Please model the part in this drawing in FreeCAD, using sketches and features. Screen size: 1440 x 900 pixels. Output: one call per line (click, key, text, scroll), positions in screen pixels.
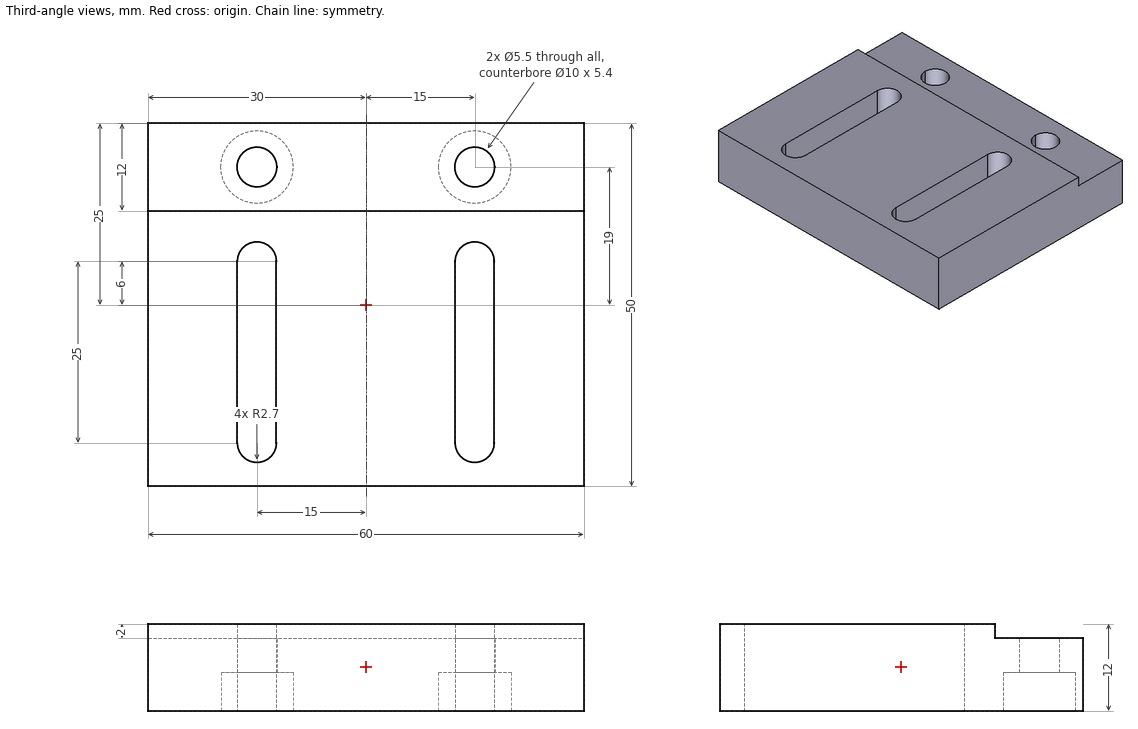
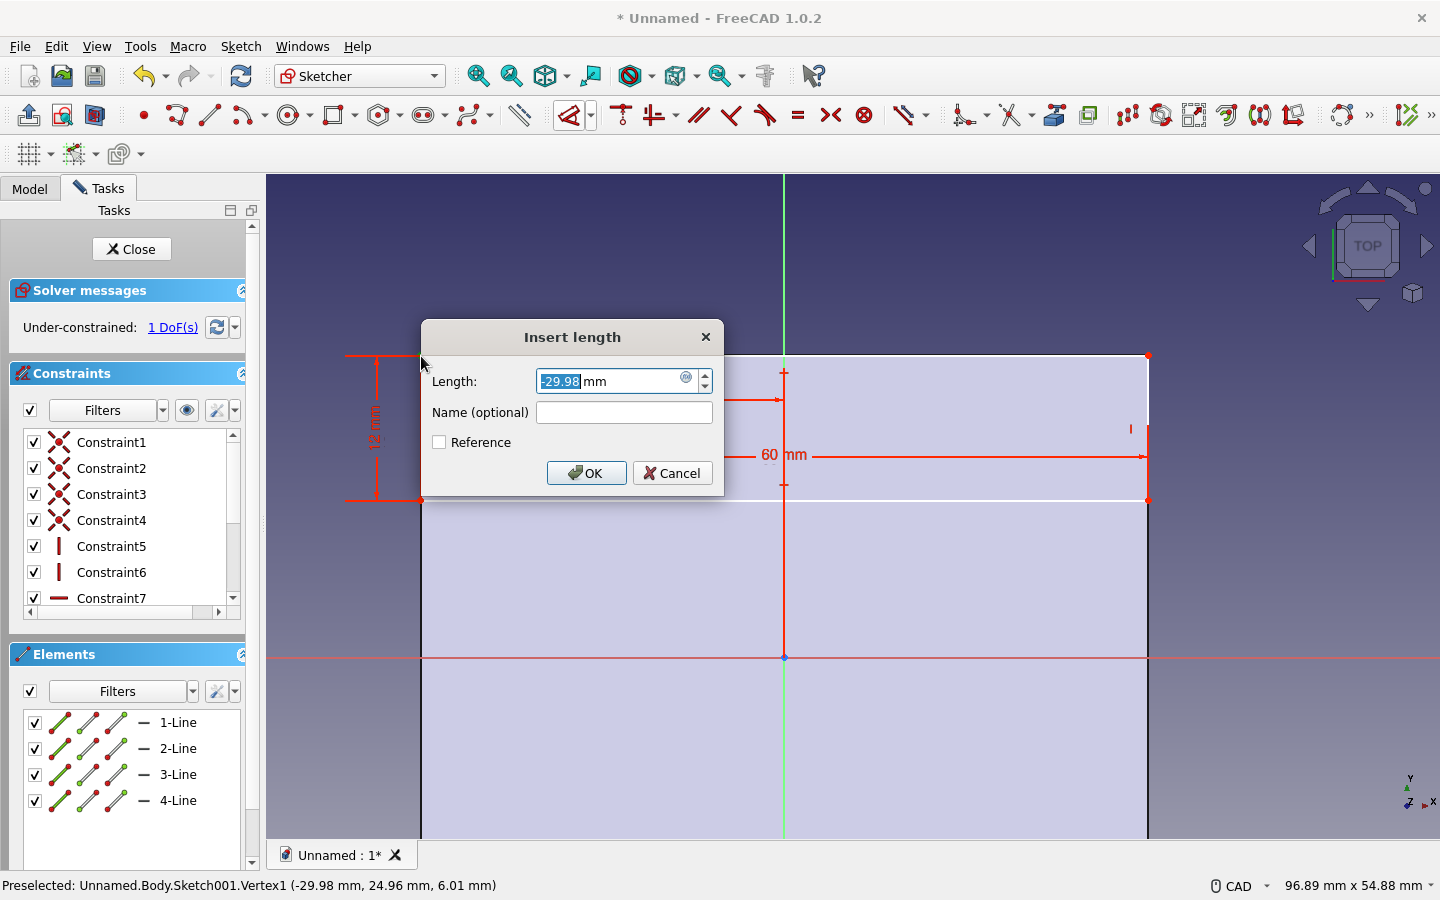
text(-30)
key(Return)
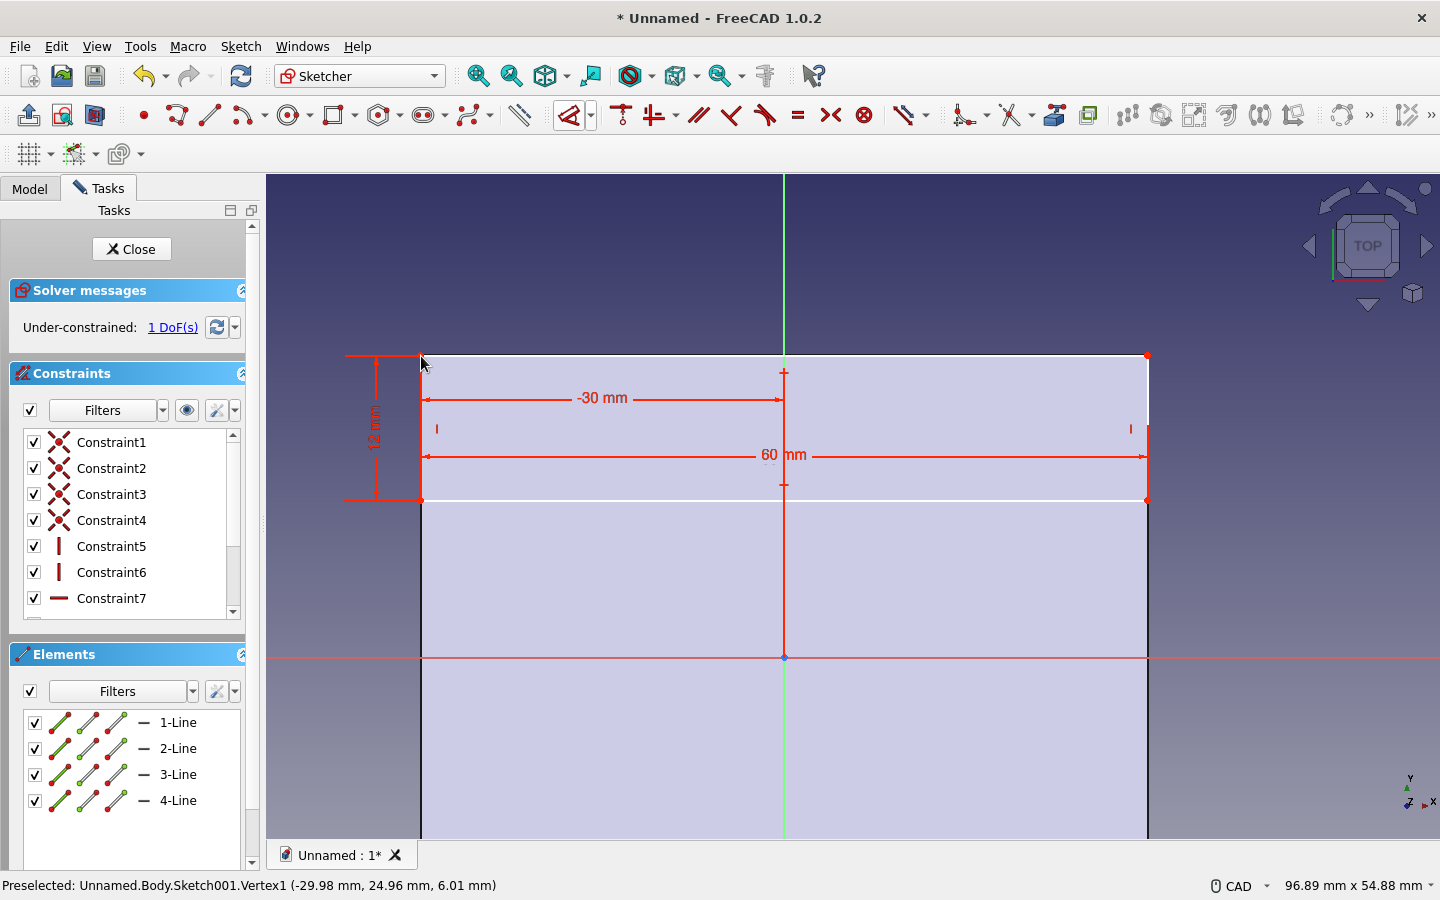
click(421, 356)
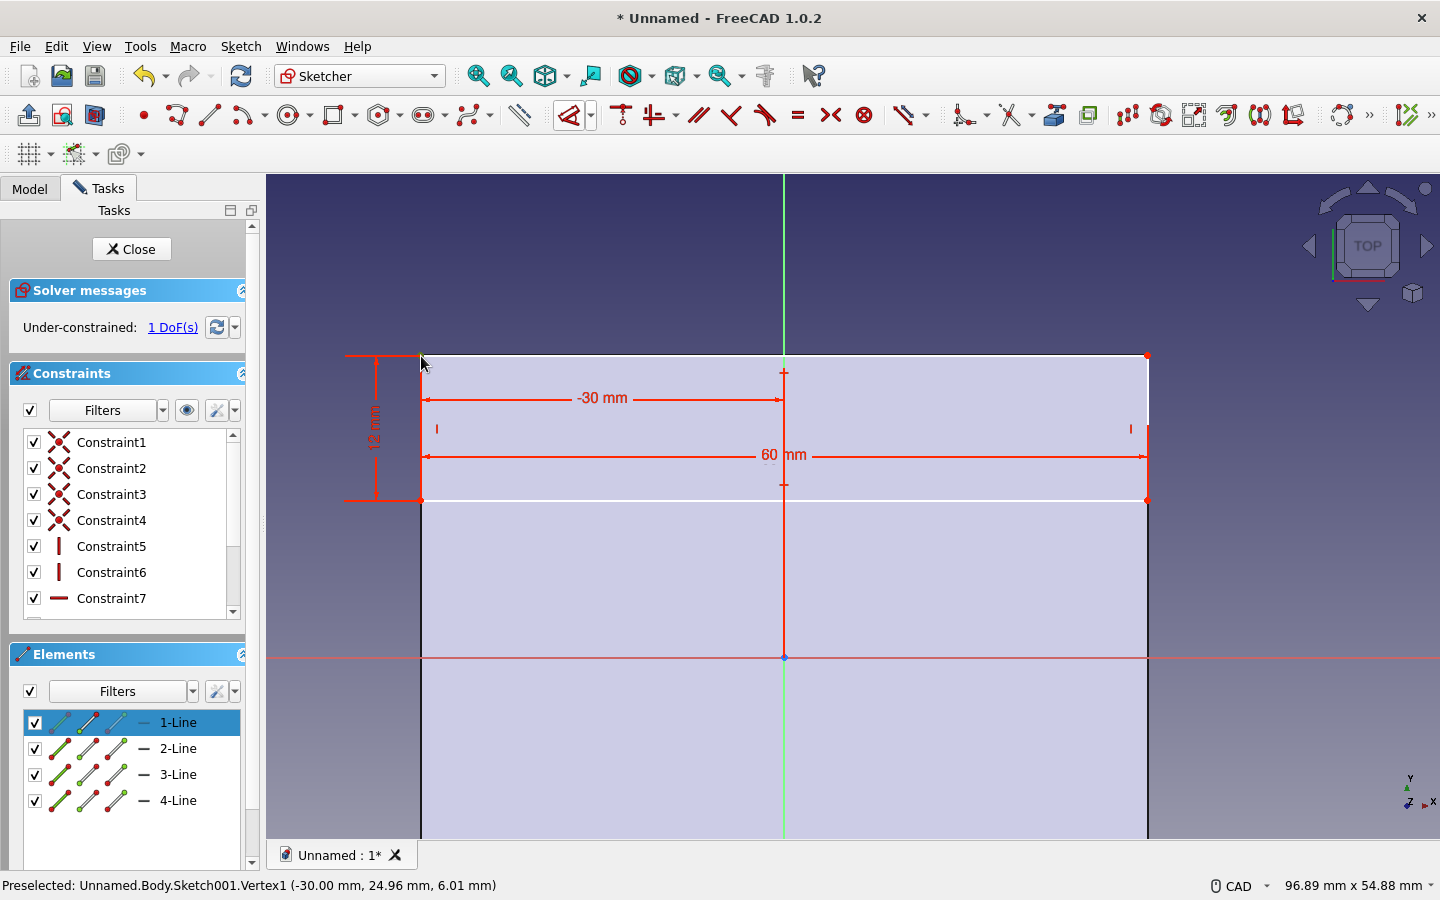
key(i)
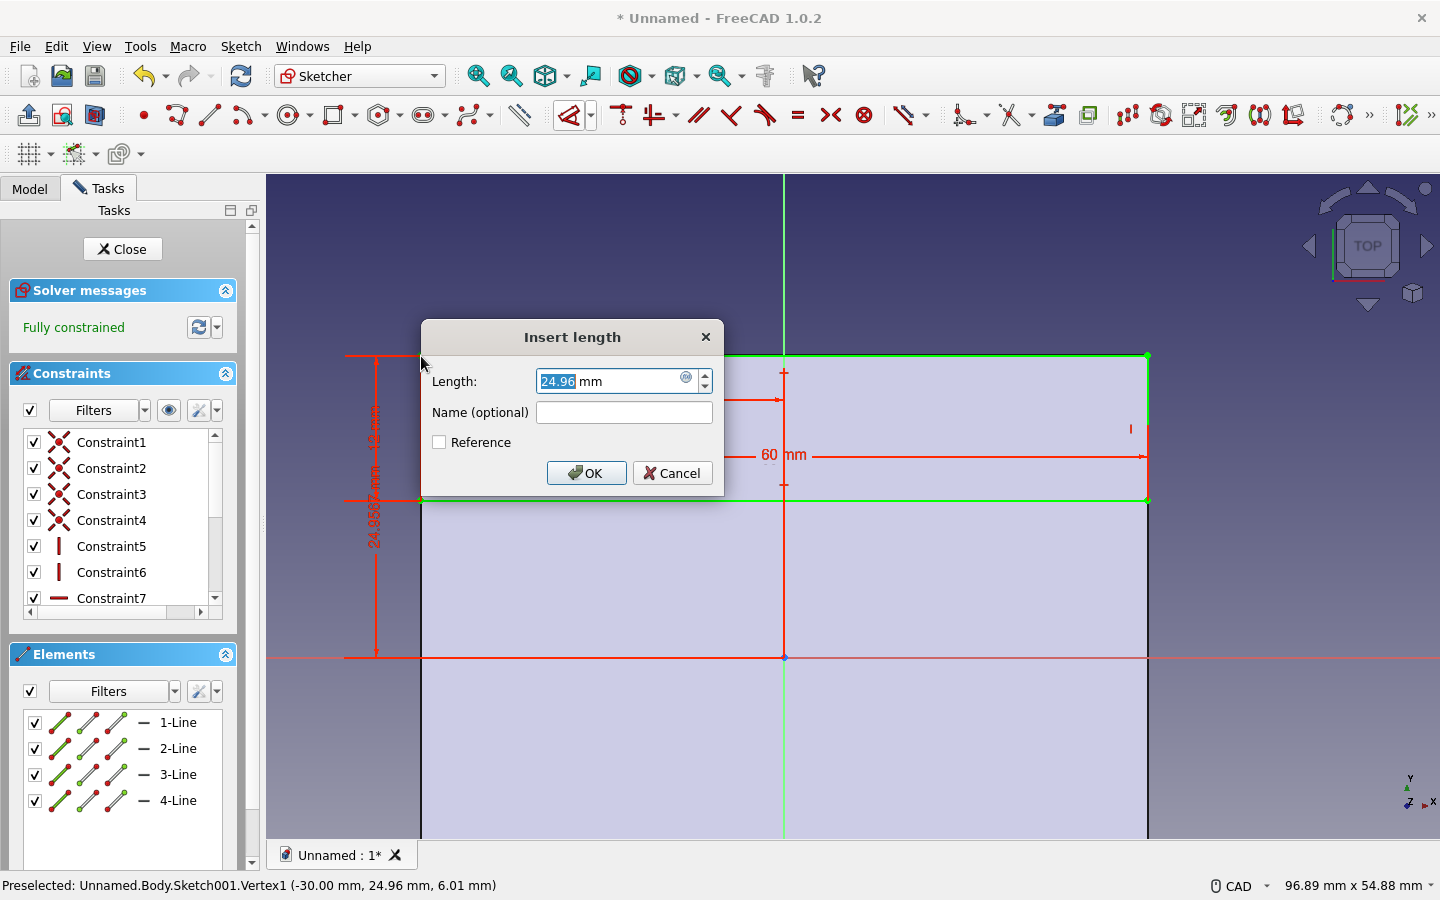
text(25)
key(Return)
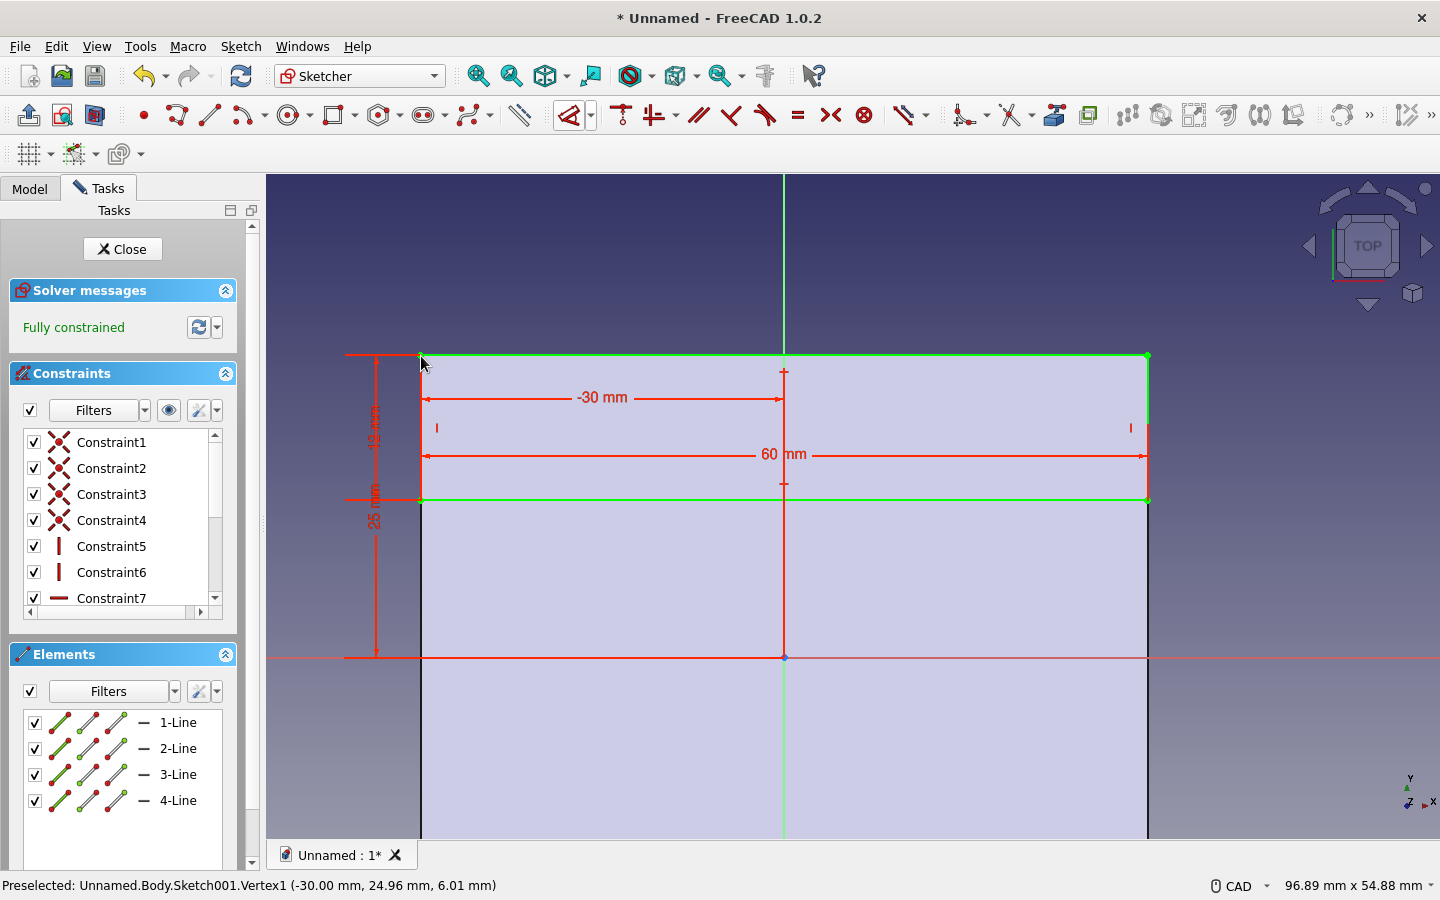
click(123, 249)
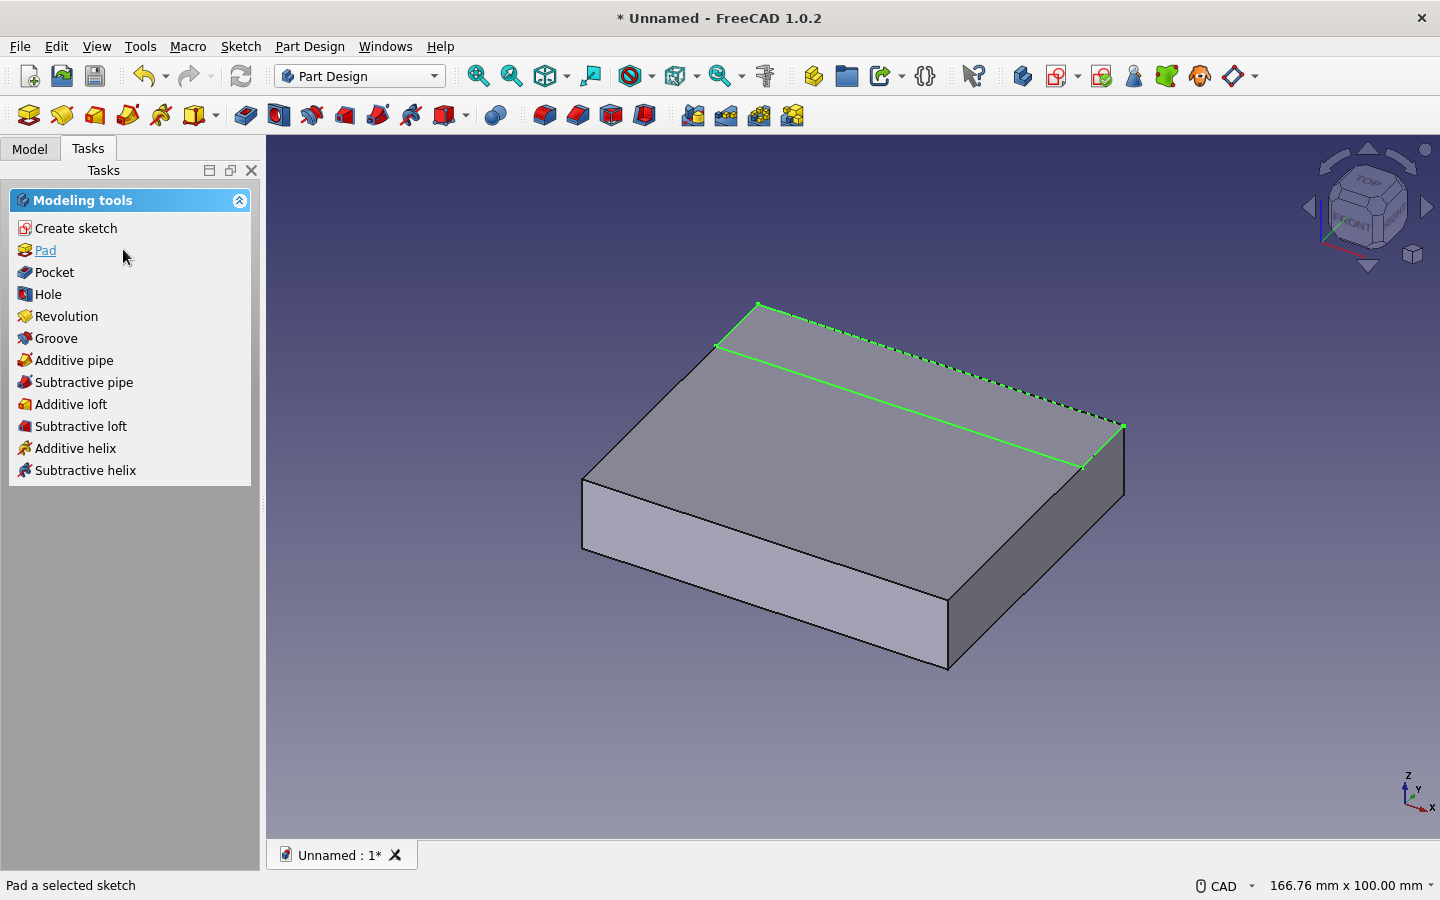
click(246, 116)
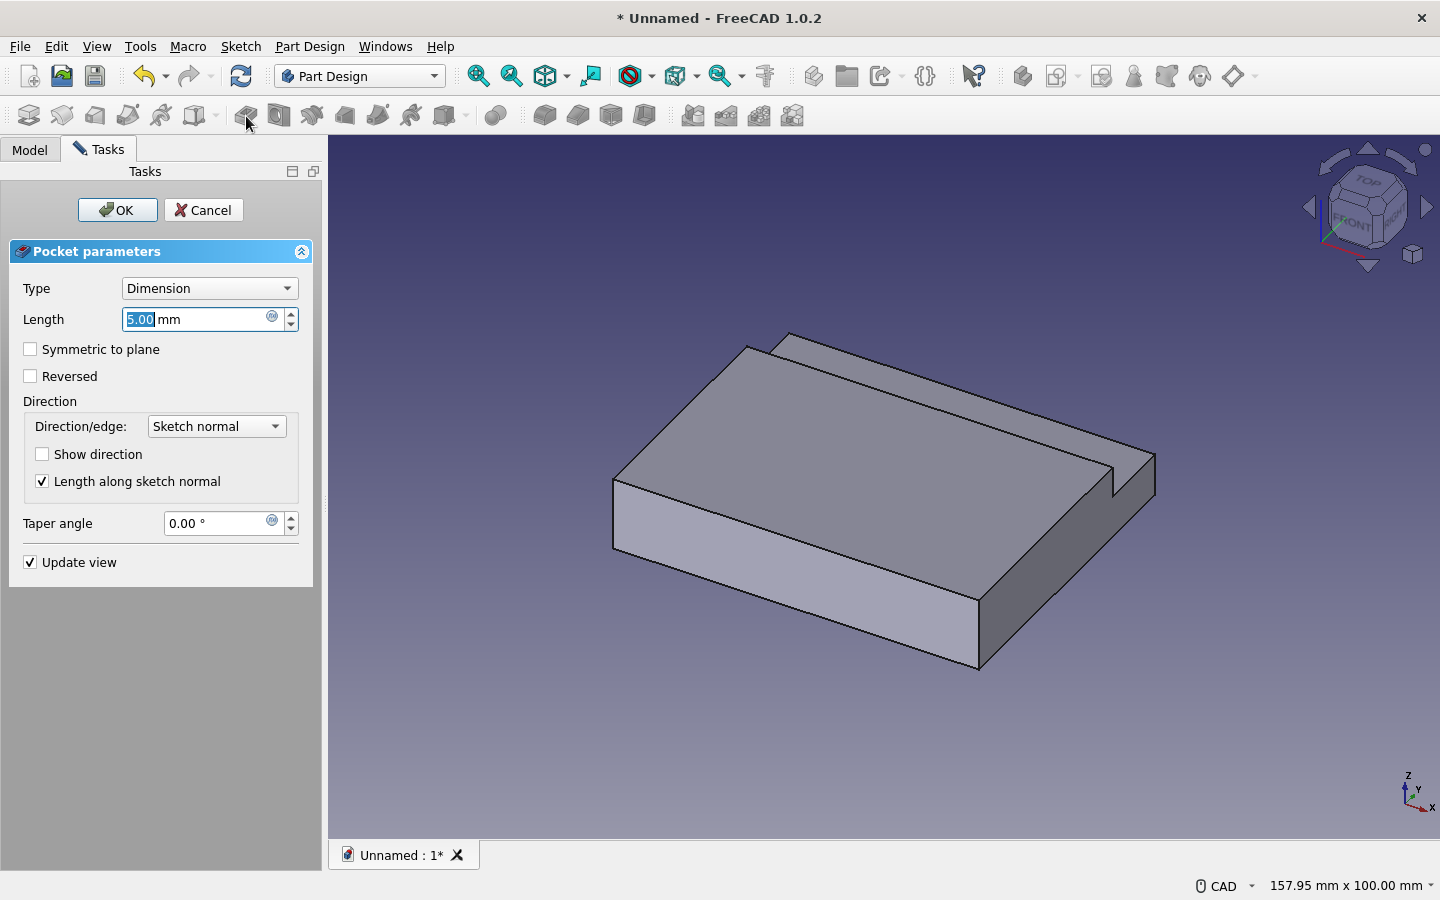
text(2)
key(Tab)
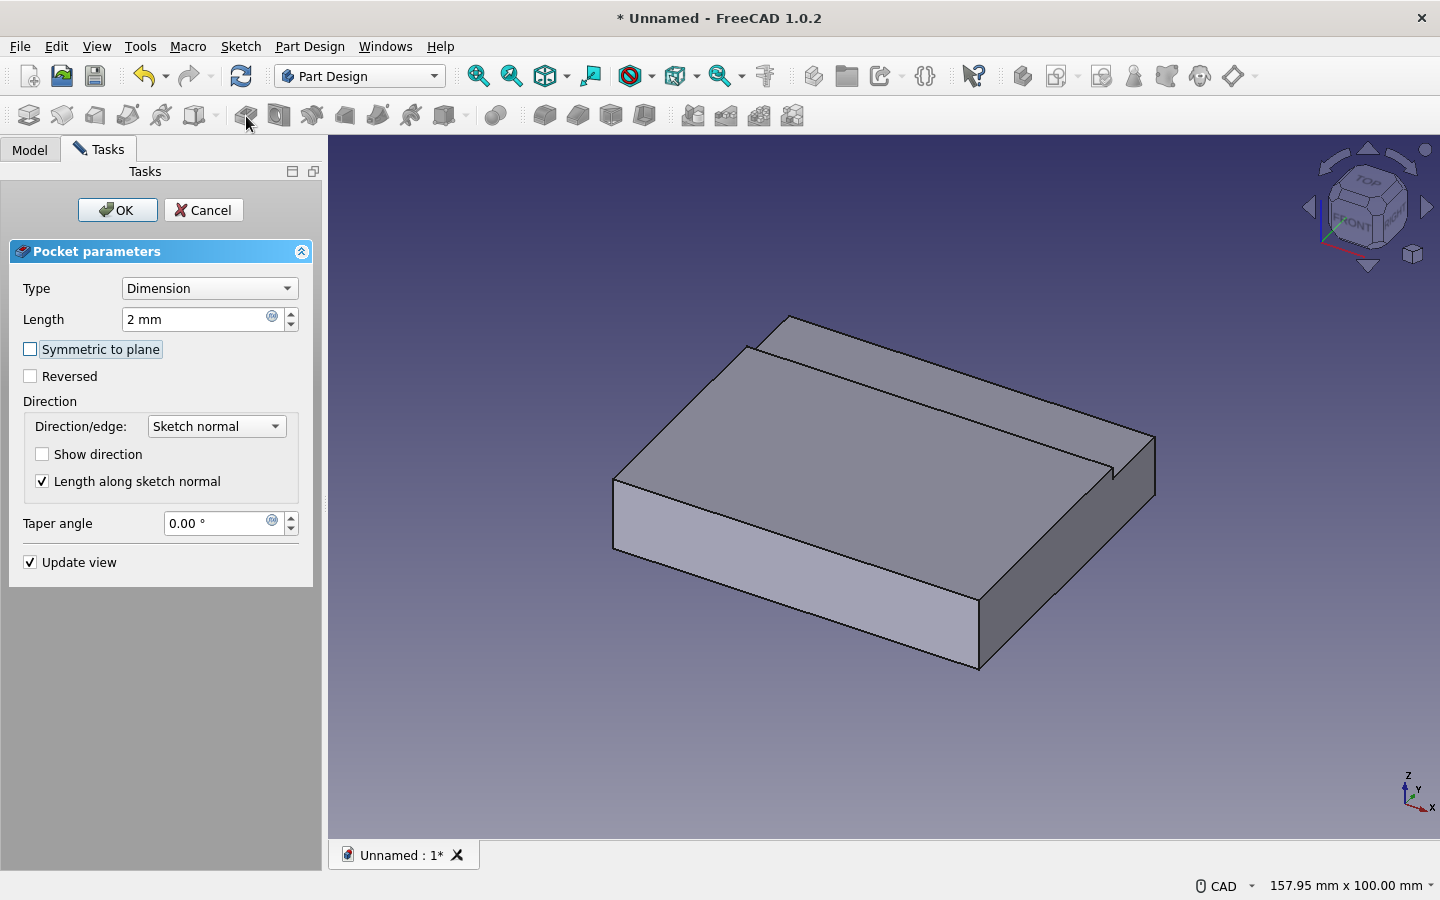
click(118, 210)